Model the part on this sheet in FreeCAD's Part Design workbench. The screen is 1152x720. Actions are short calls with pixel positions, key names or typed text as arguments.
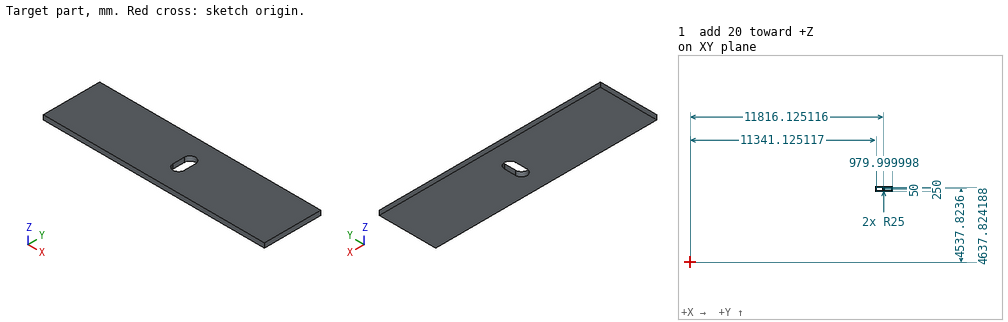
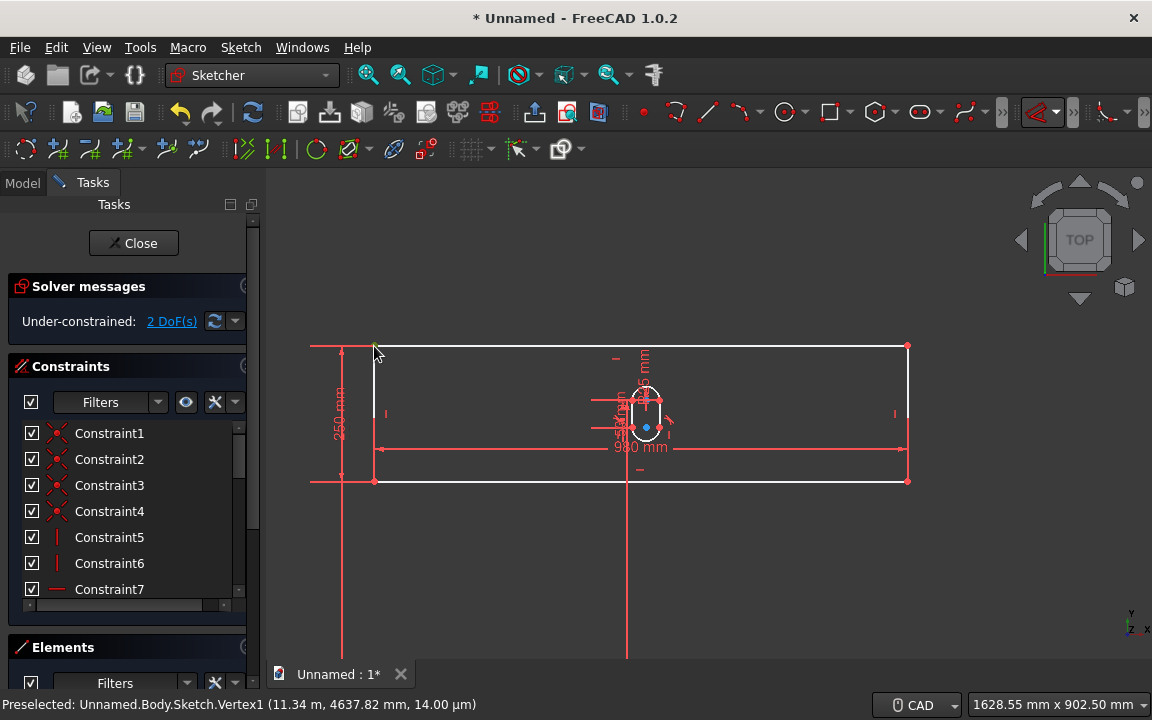
click(1058, 112)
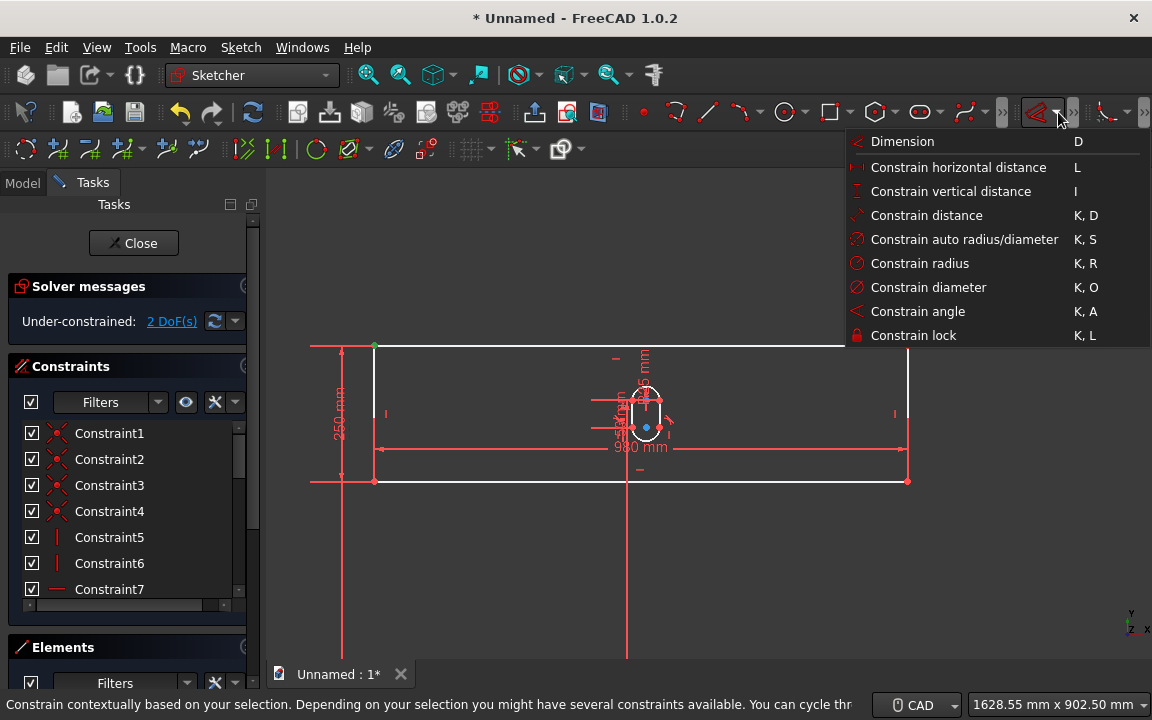
click(998, 167)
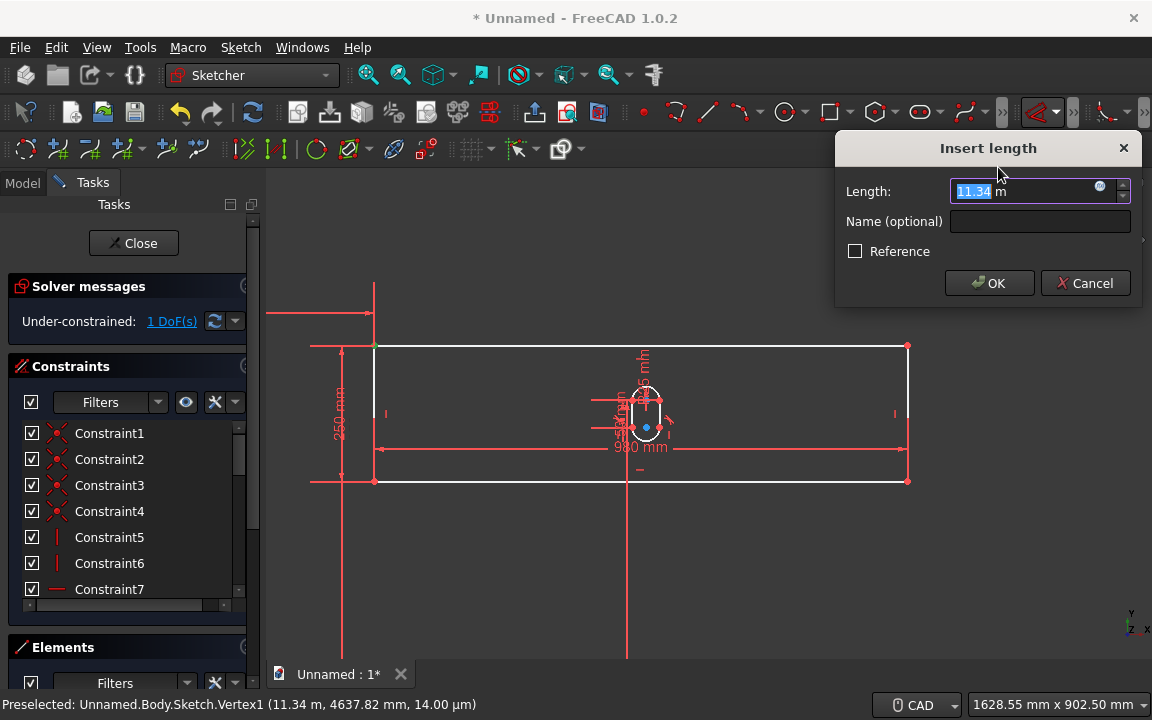
key(ctrl+a)
text(11341.125117 mm)
key(Return)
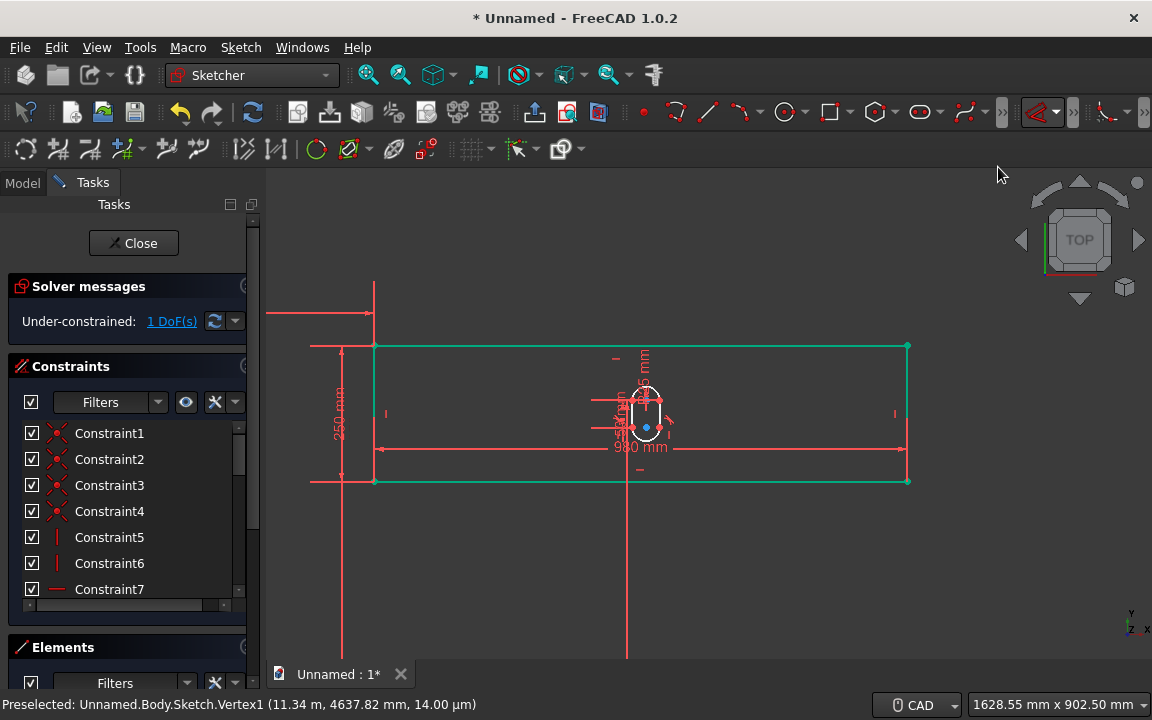
click(632, 428)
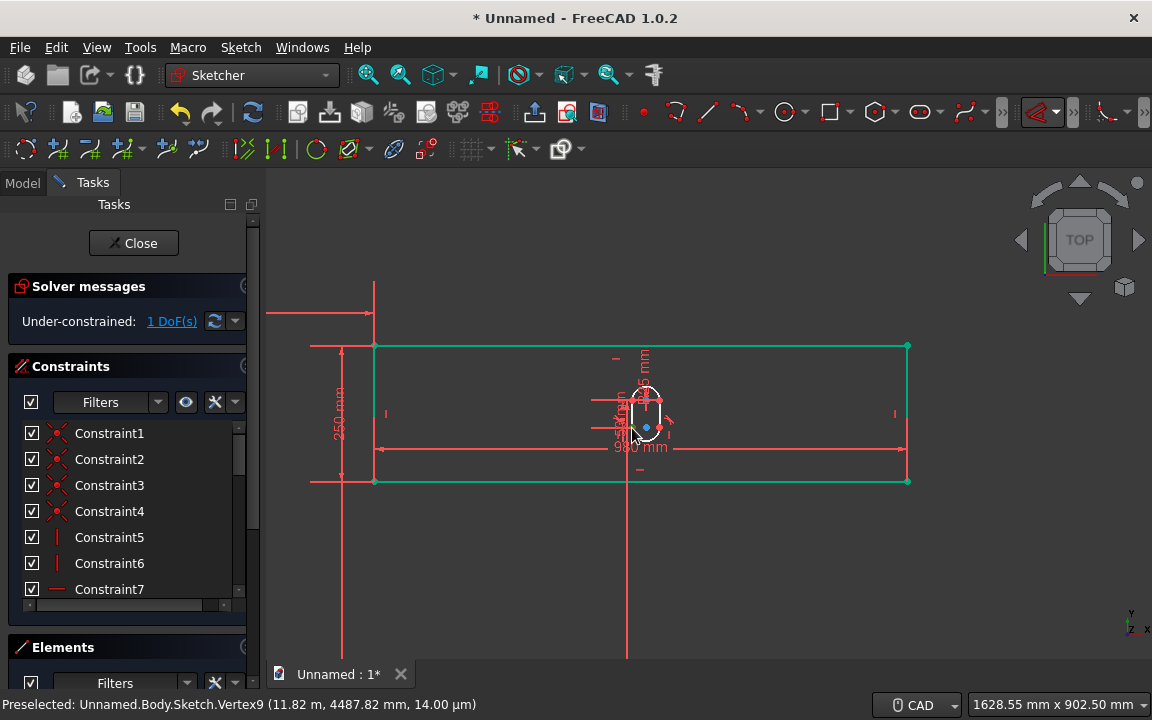
click(1058, 112)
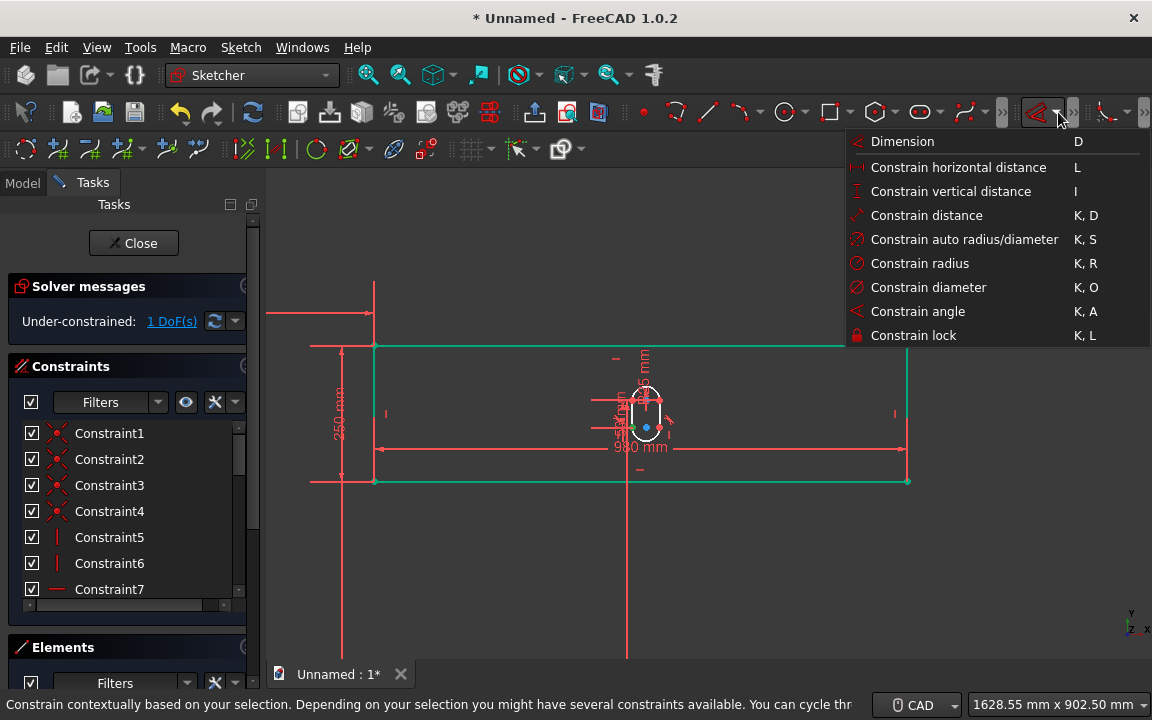
click(998, 167)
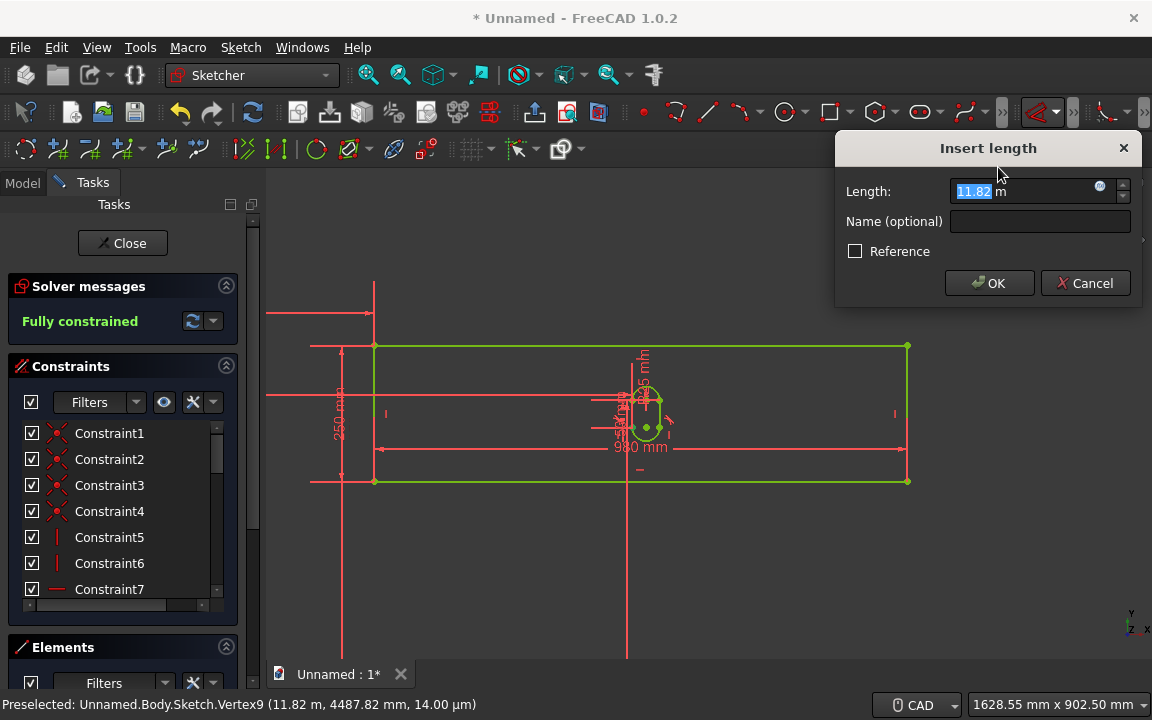
key(ctrl+a)
text(11816.125116 mm)
key(Return)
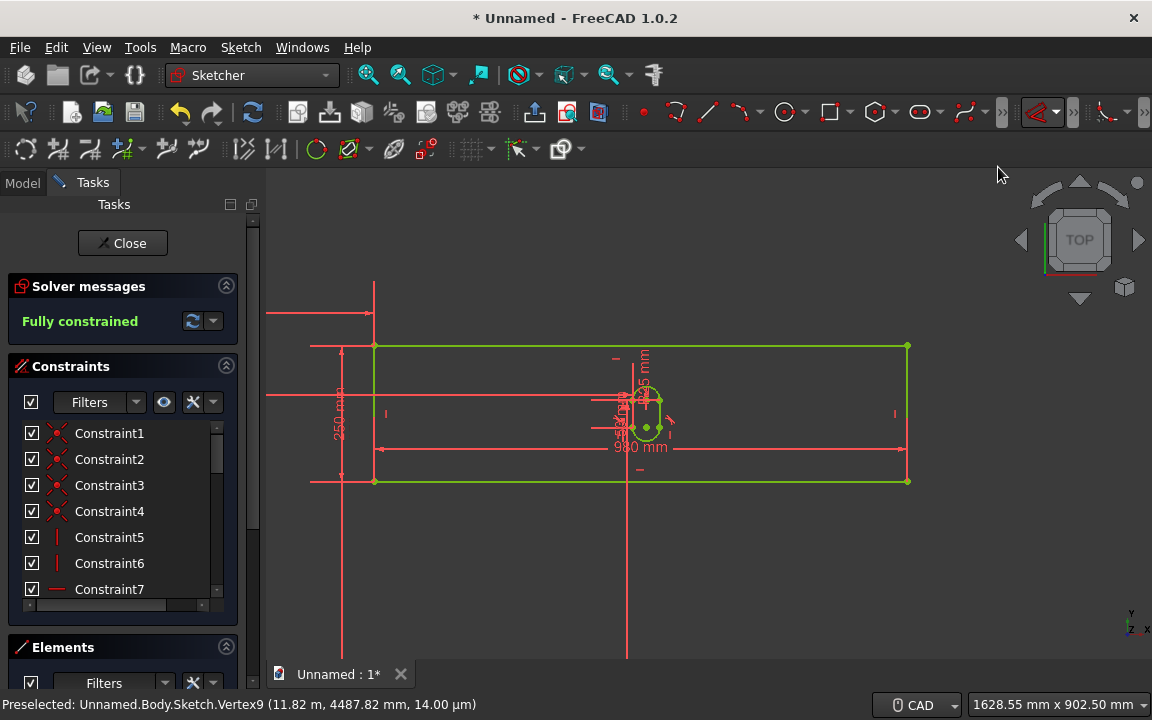
click(123, 243)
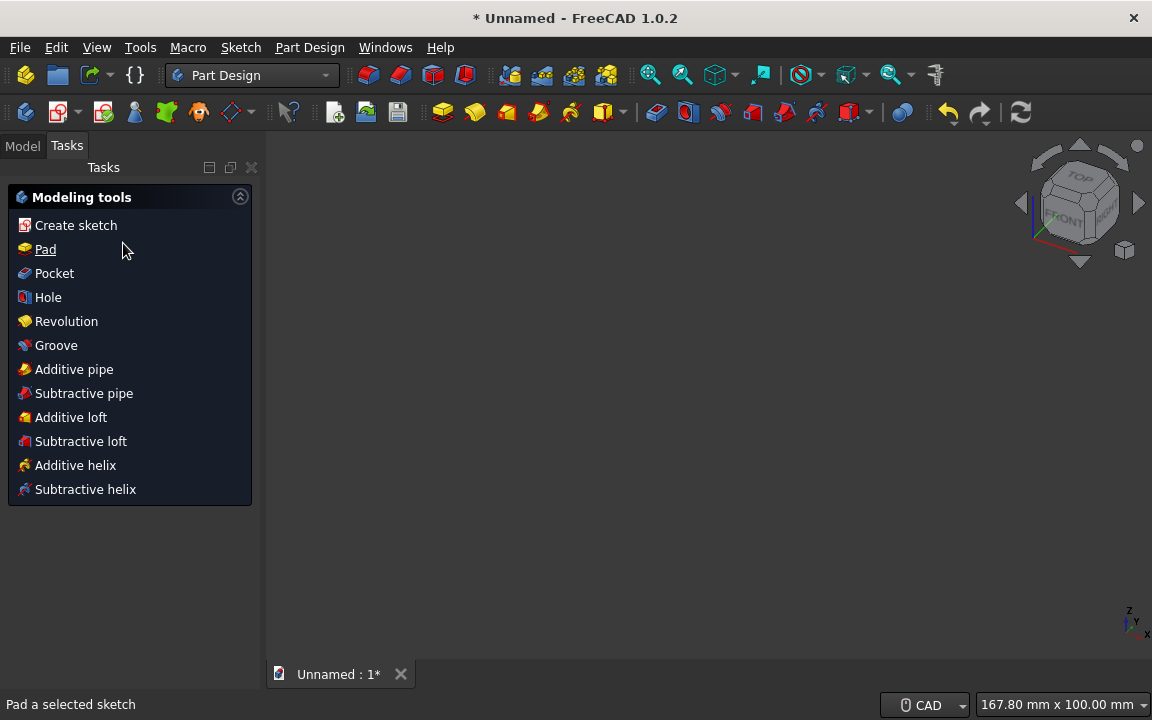
click(444, 112)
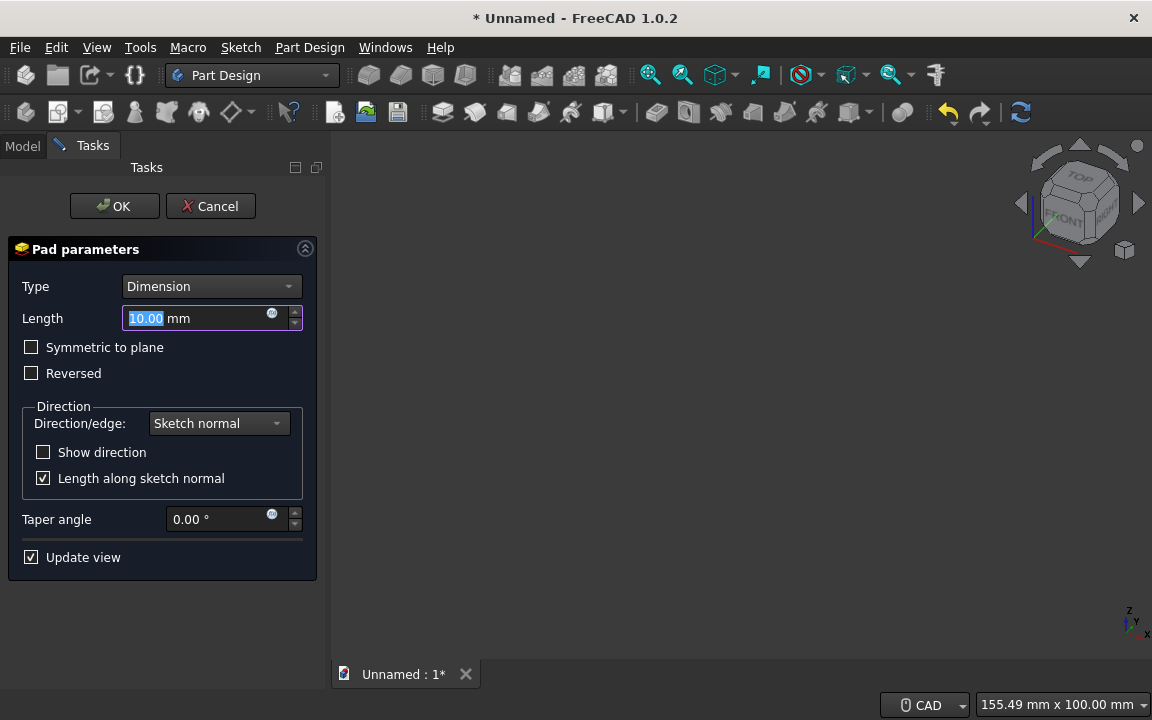
text(20)
key(Tab)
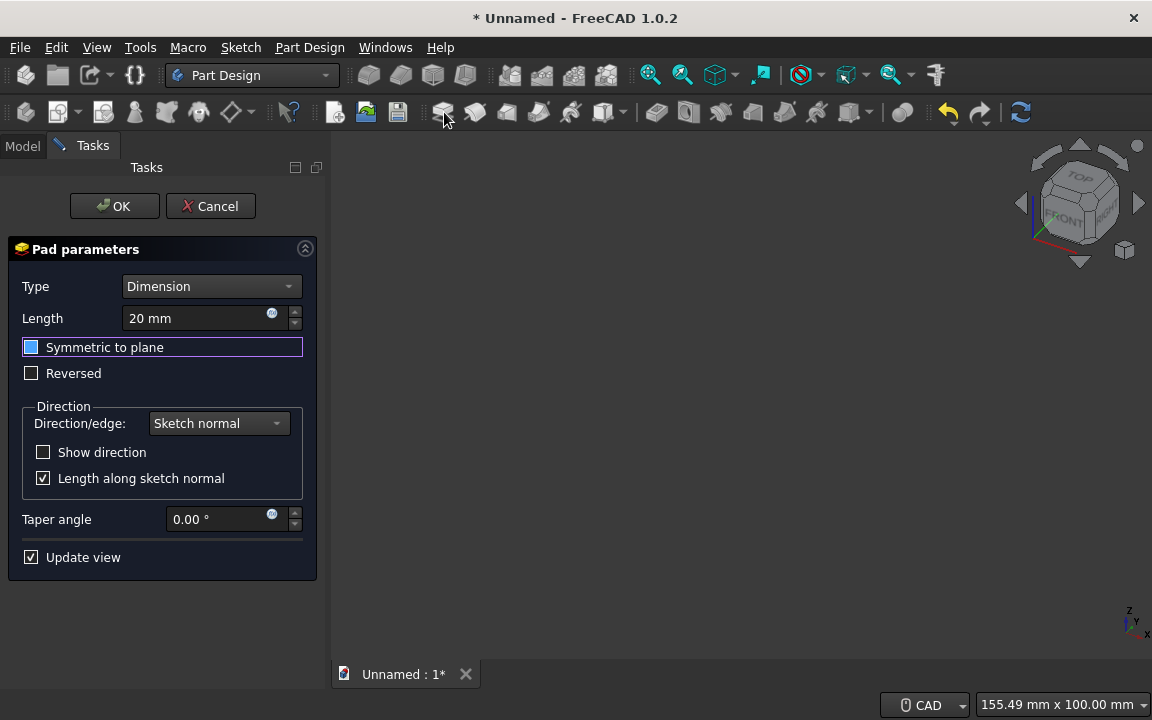
click(115, 206)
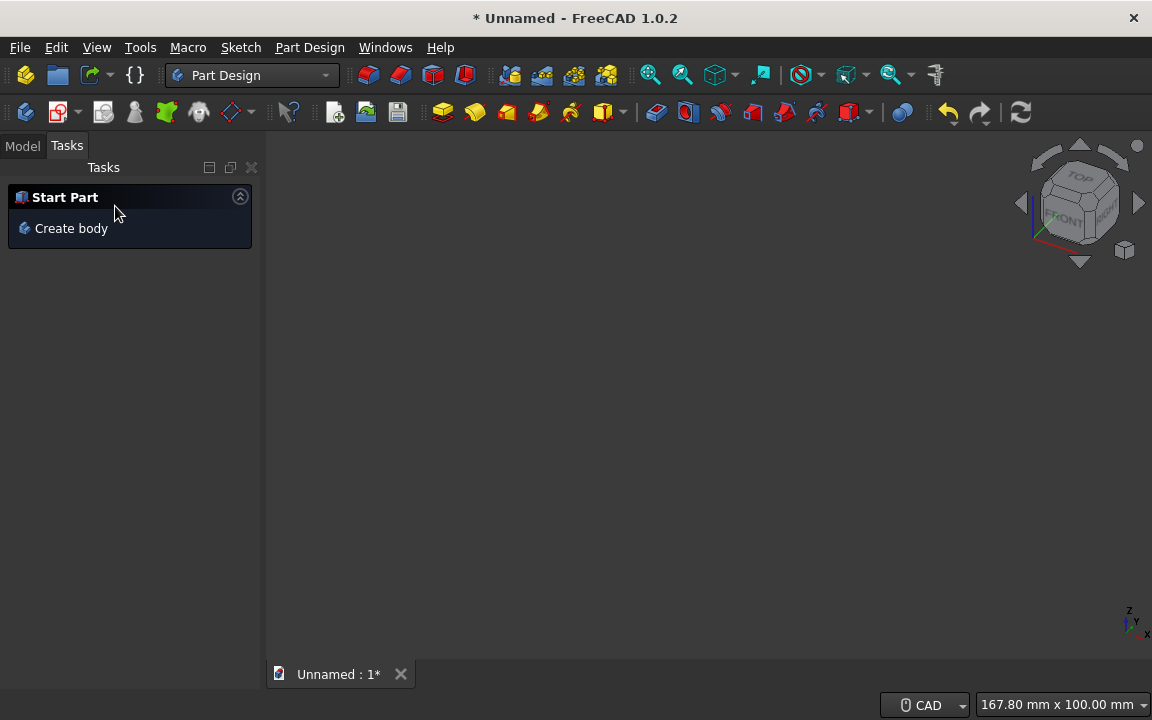
key(0)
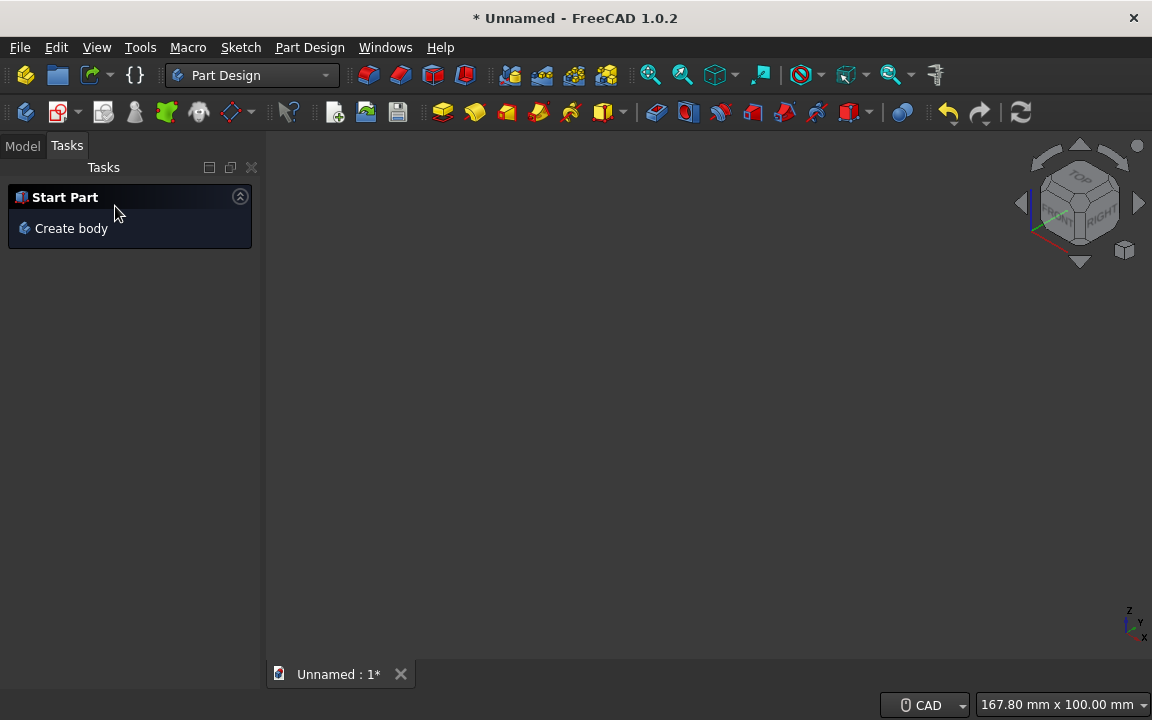
key(v)
key(f)